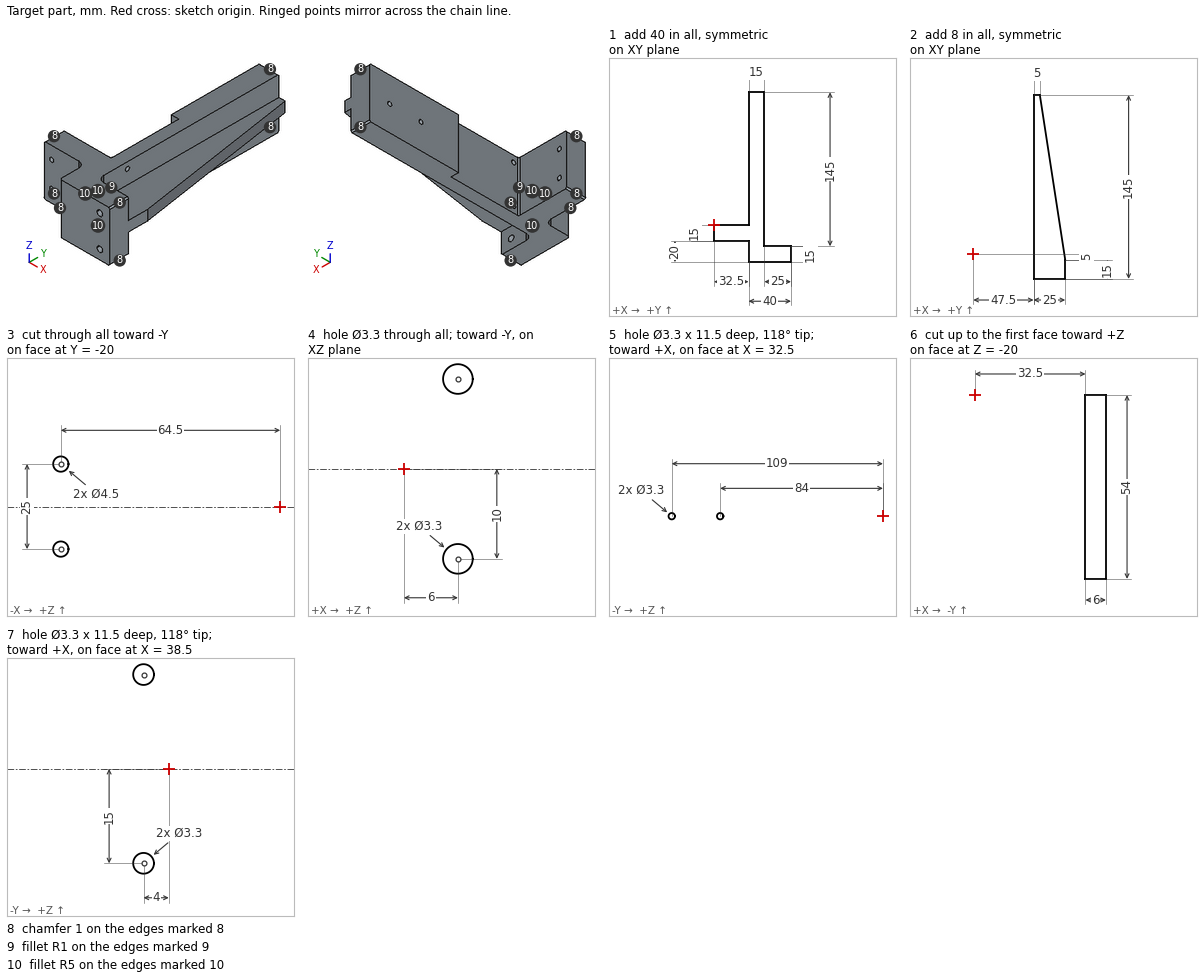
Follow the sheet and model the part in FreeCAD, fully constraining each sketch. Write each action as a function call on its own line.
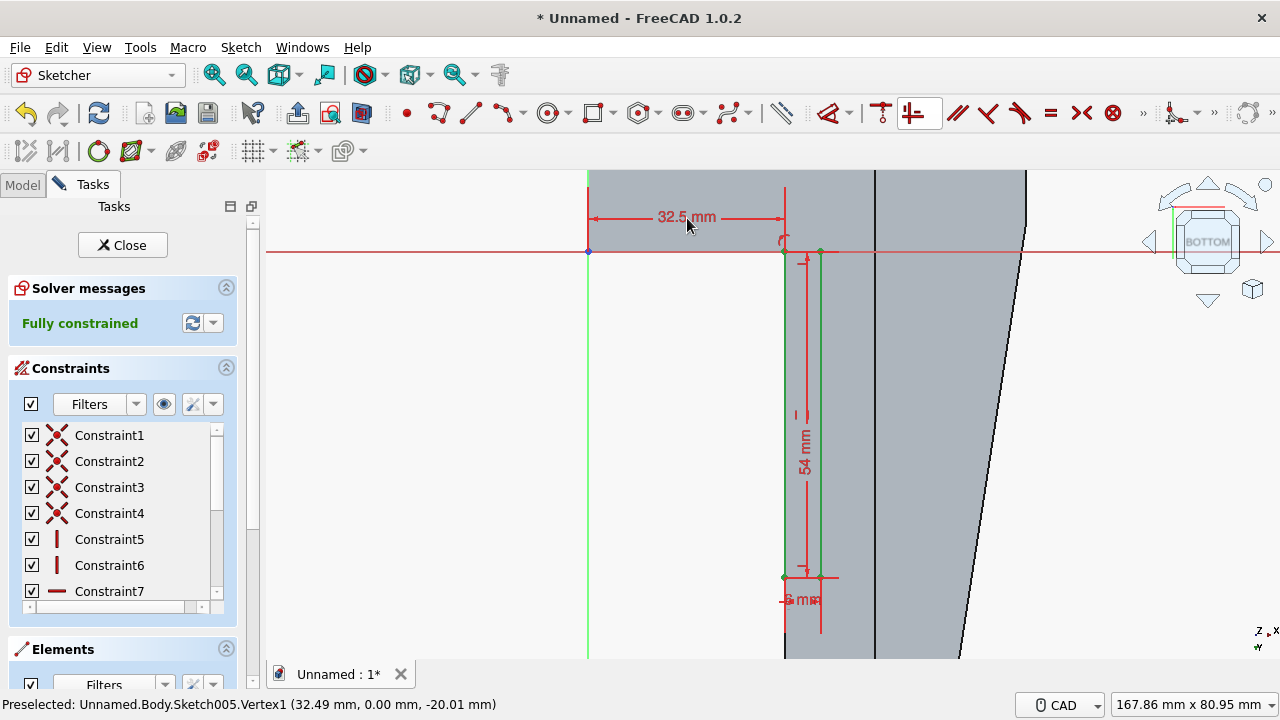
click(123, 245)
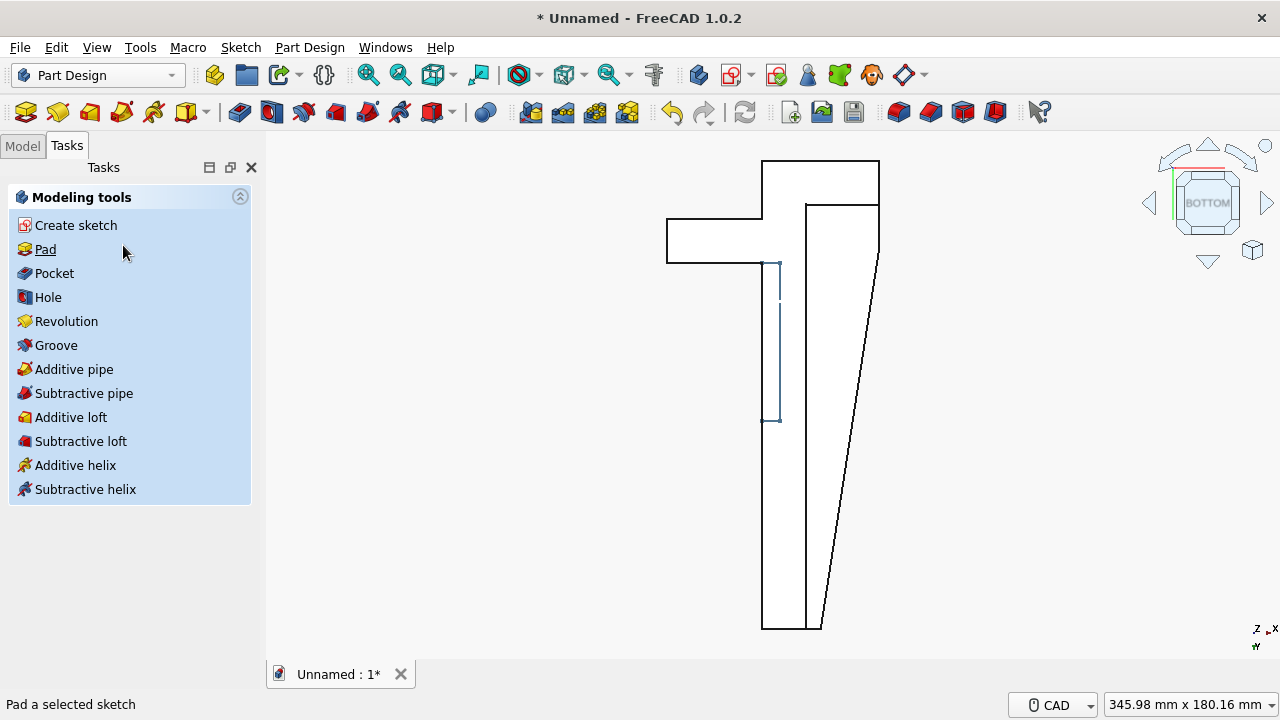
click(240, 112)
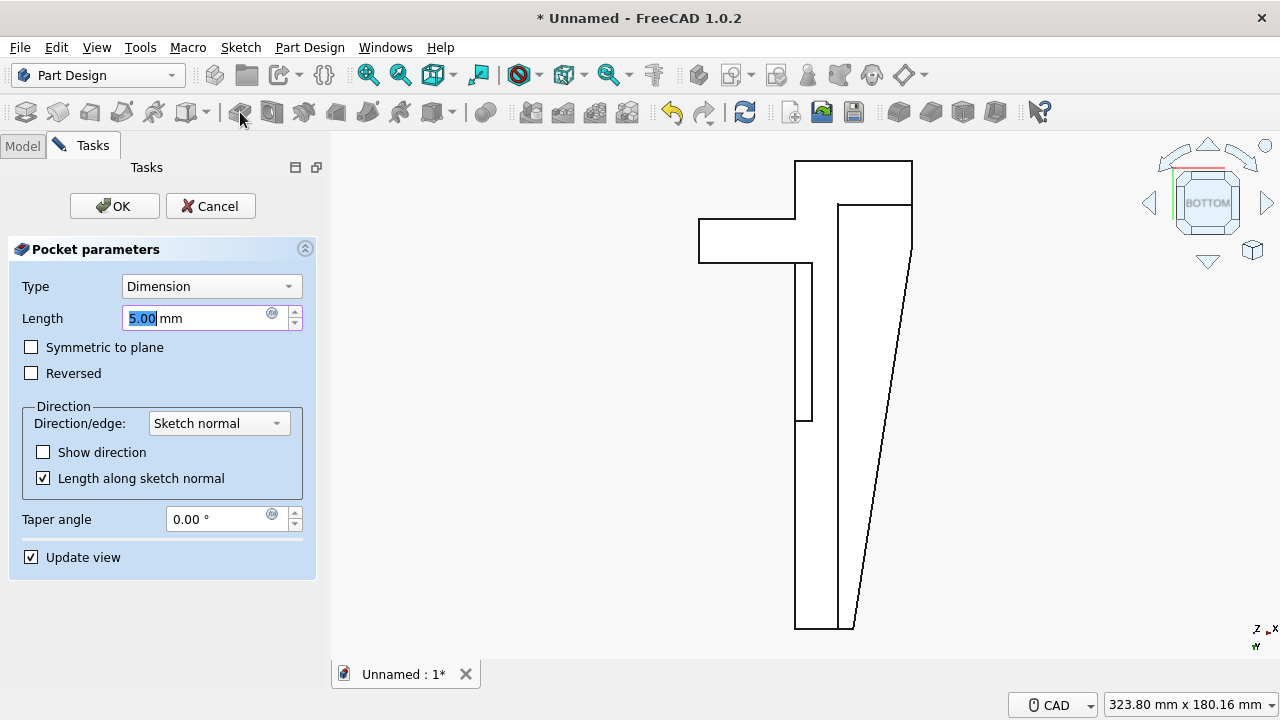
click(212, 286)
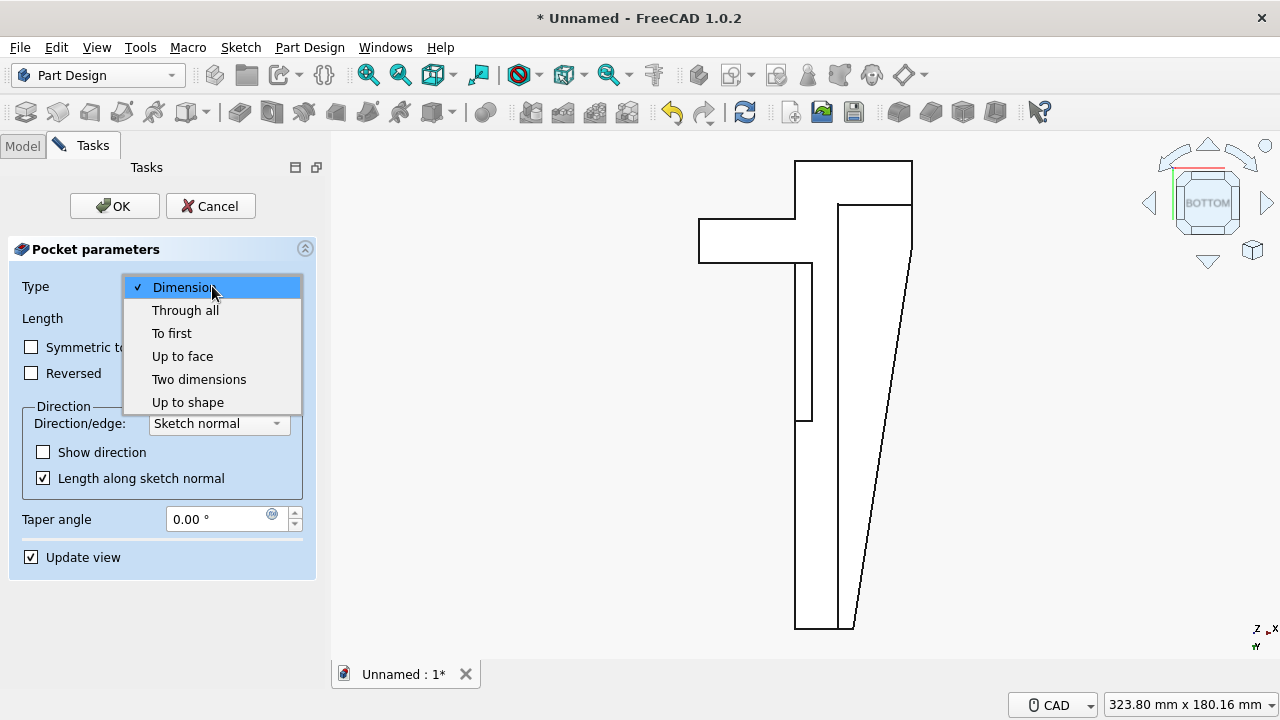
click(212, 334)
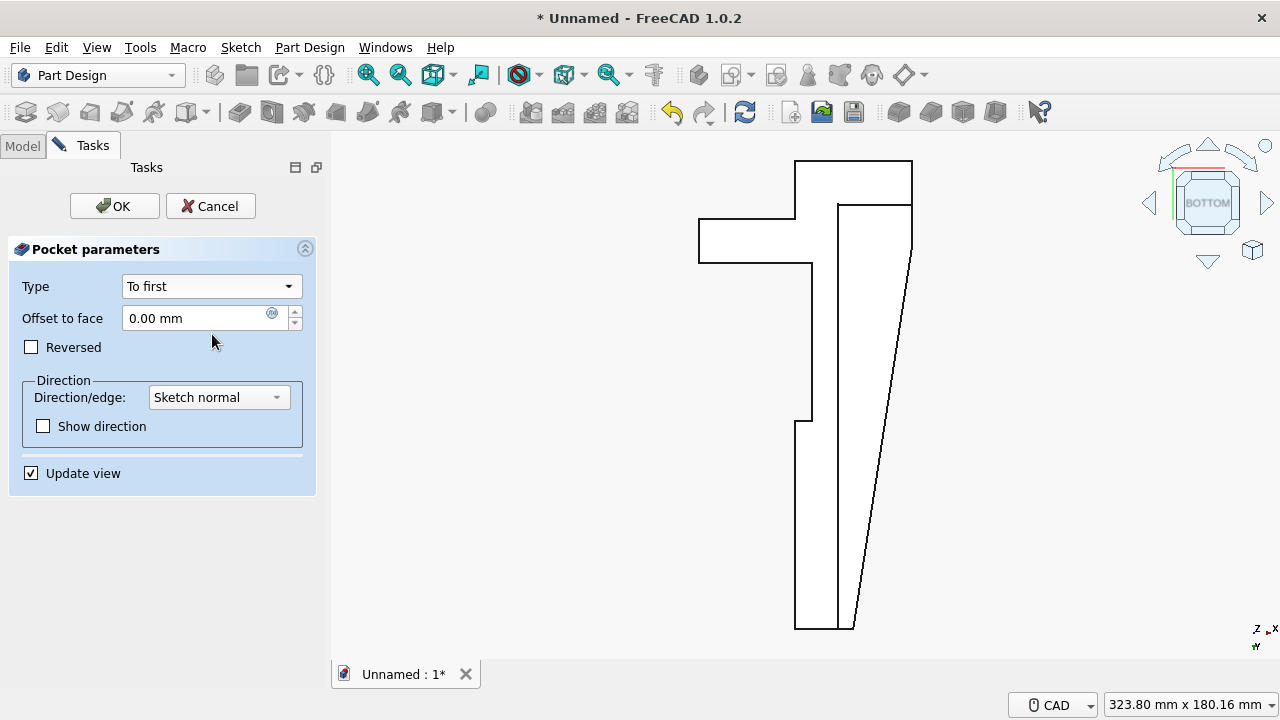
click(115, 206)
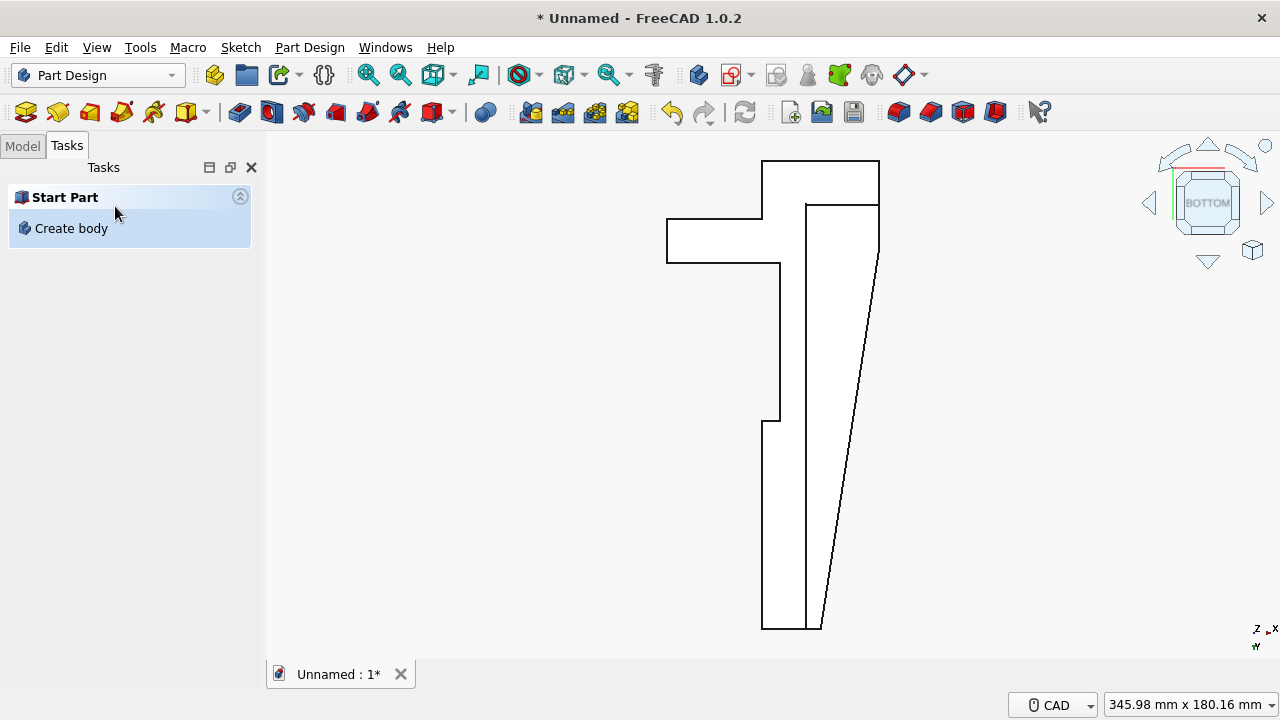
key(6)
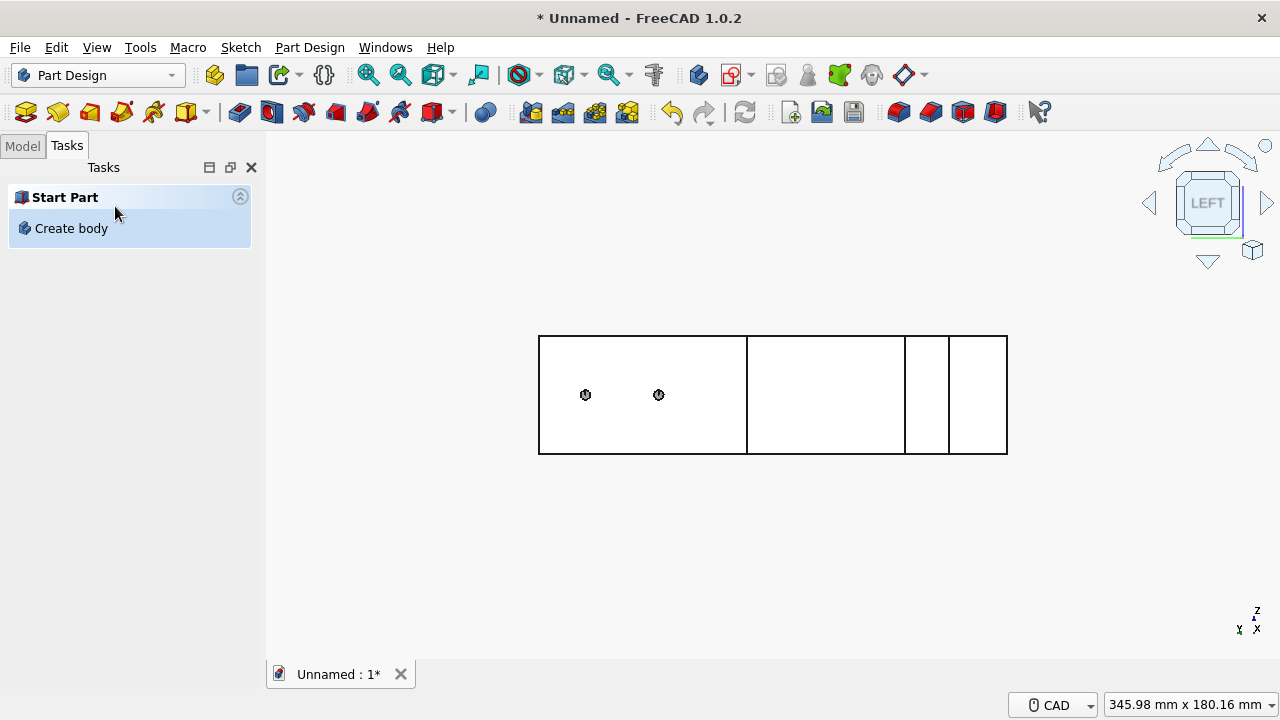
click(826, 394)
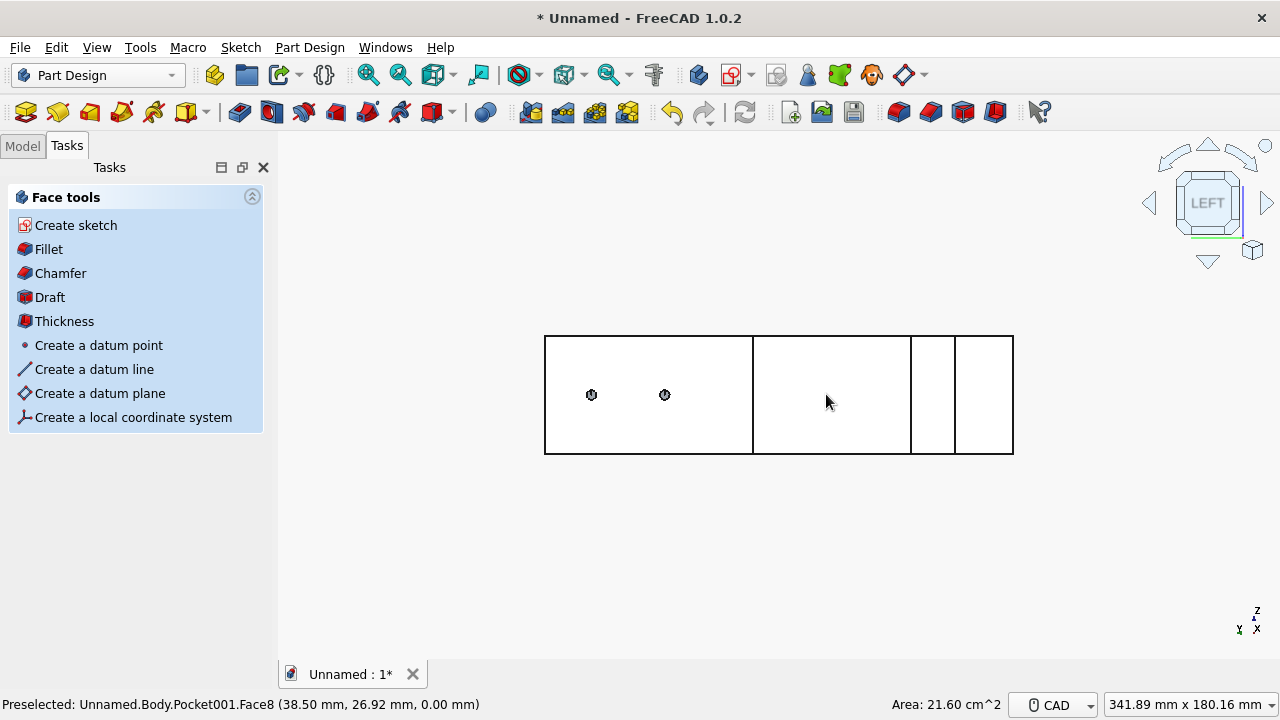
click(732, 76)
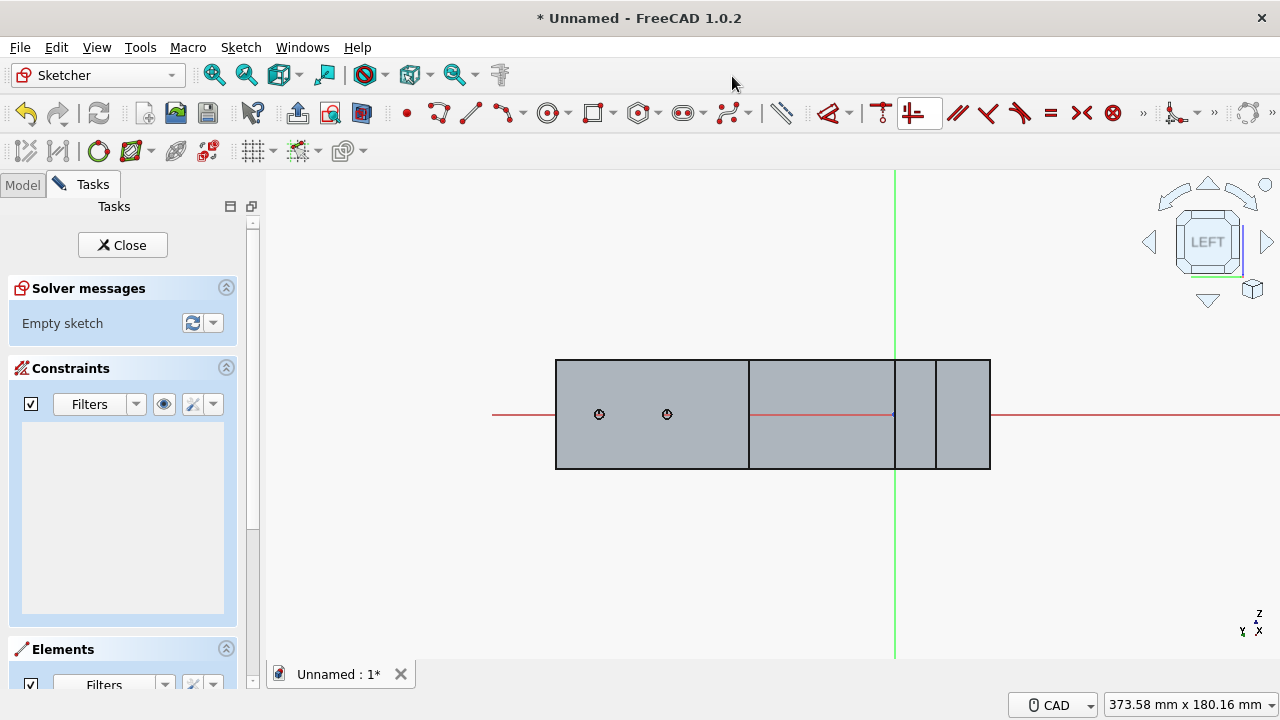
key(q)
key(s)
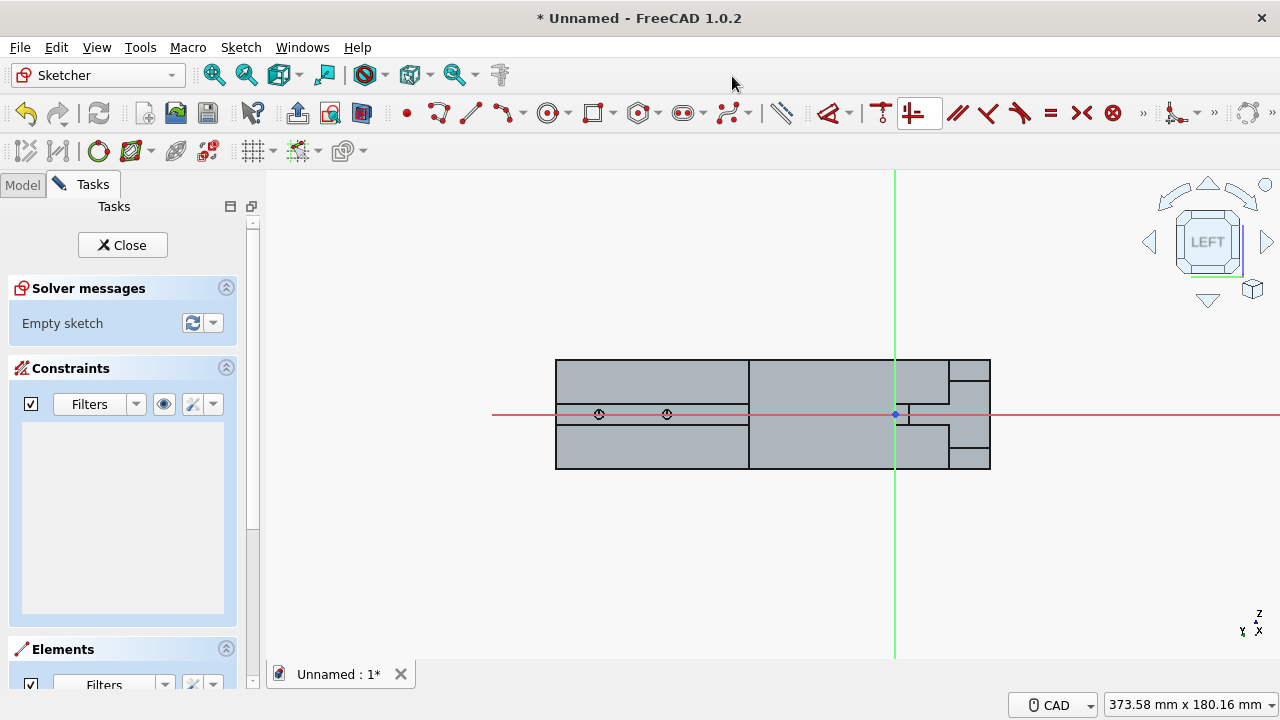
scroll(966, 415, up, 6)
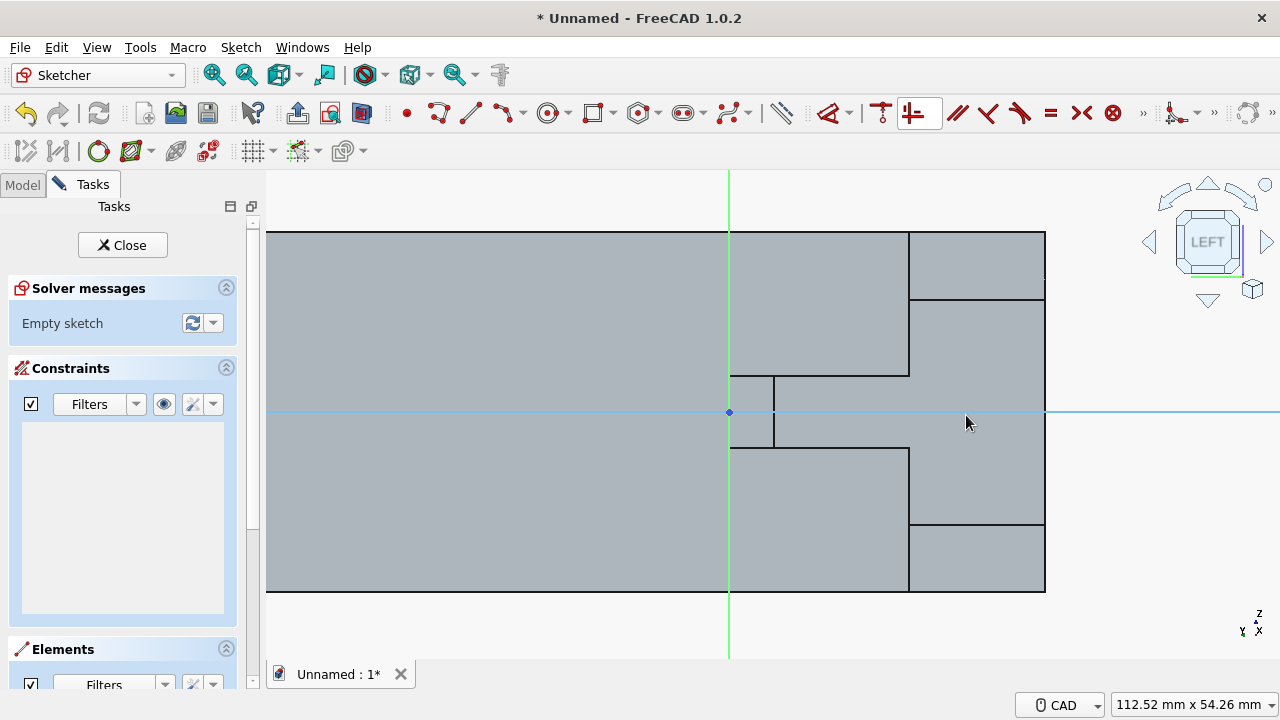
click(548, 114)